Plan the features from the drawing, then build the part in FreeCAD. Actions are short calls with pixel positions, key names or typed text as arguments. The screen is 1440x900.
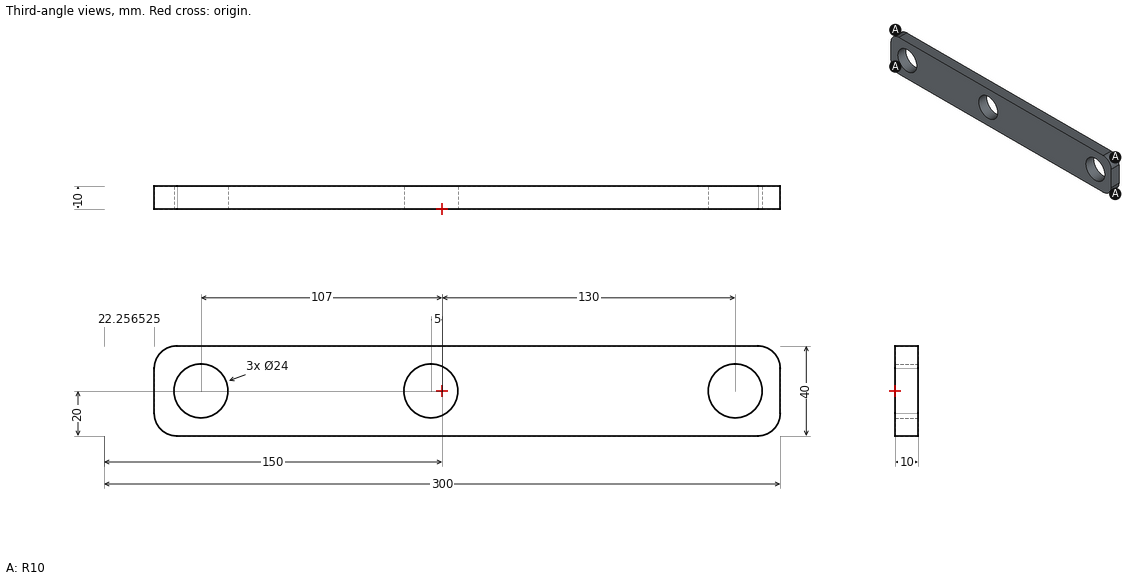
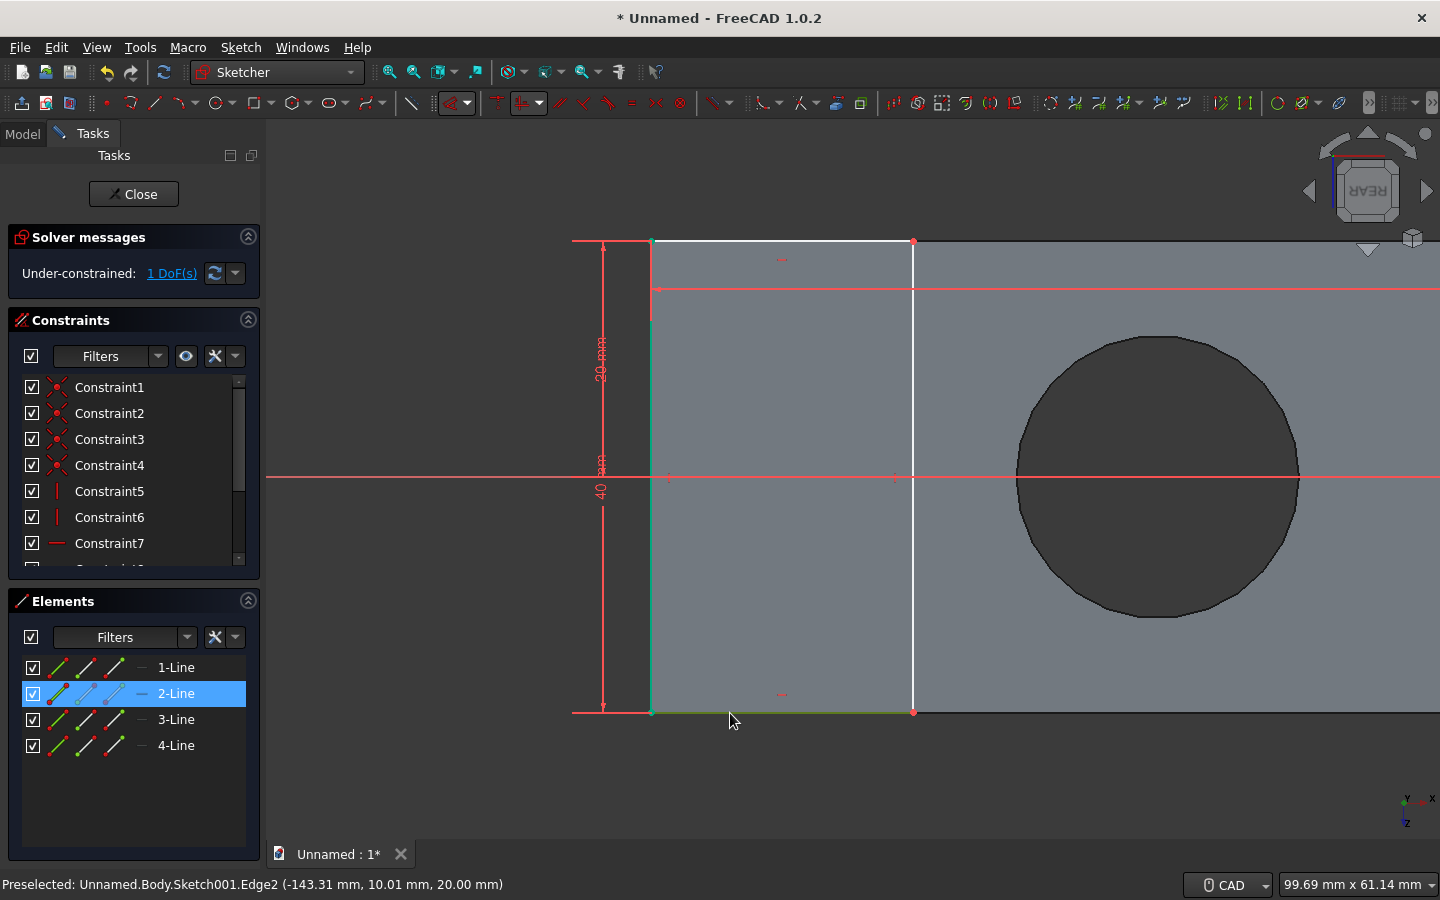
click(470, 104)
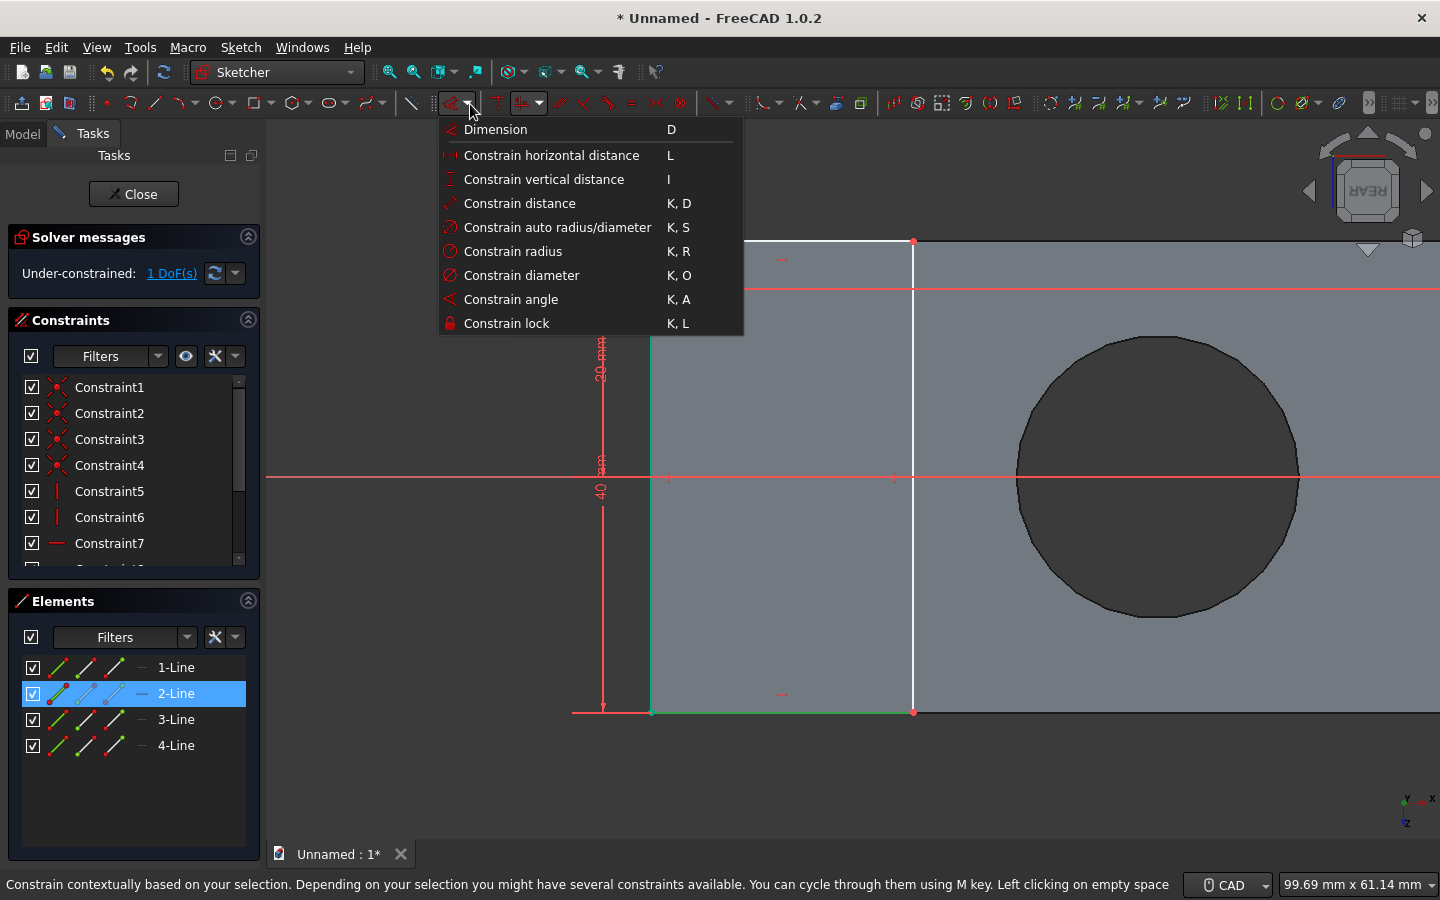
click(591, 155)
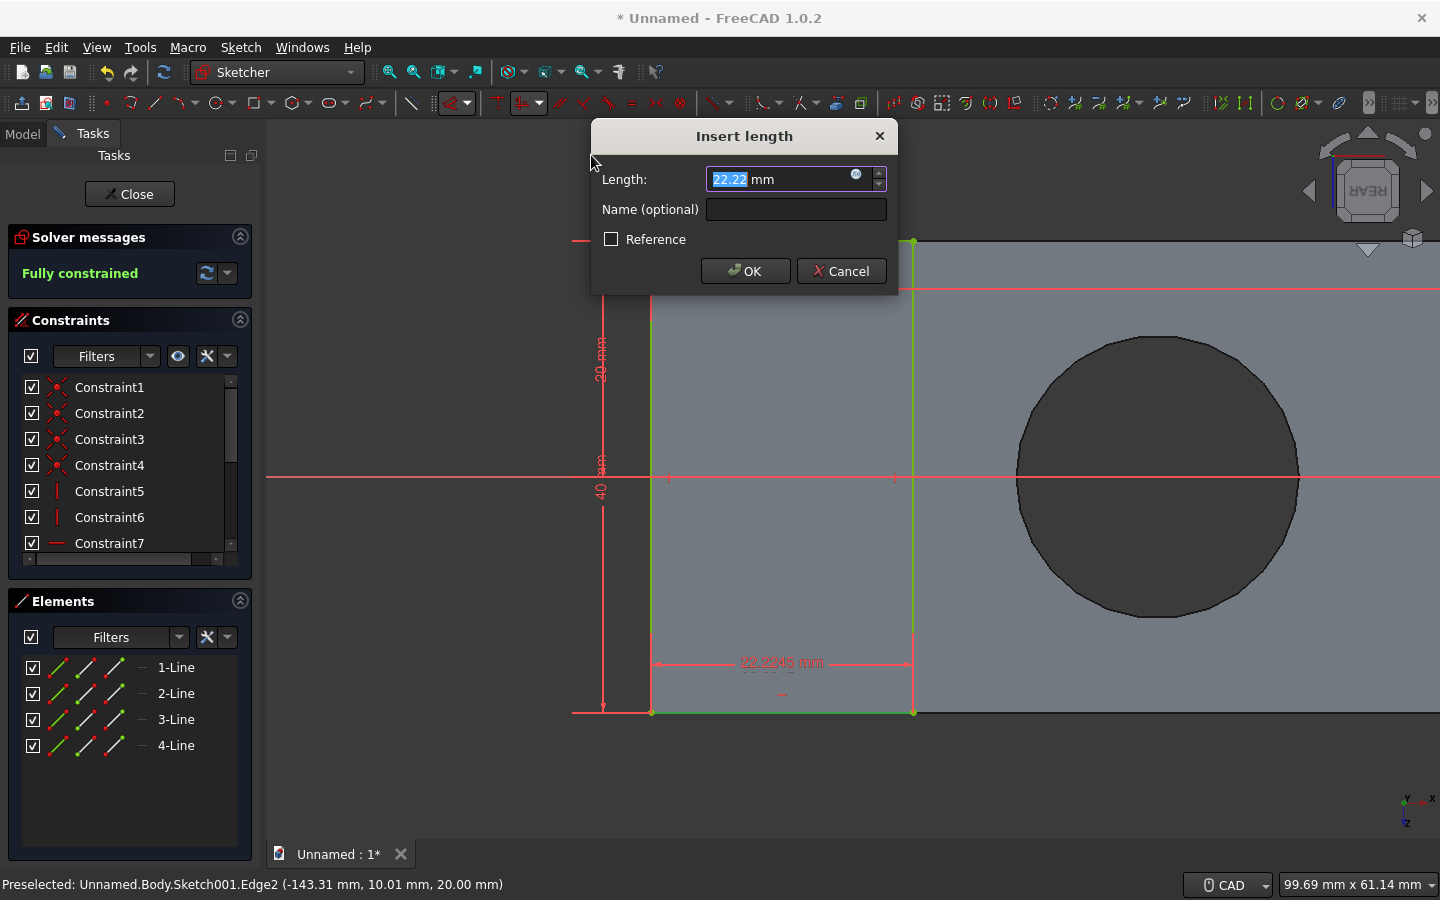
text(22.256525)
key(Return)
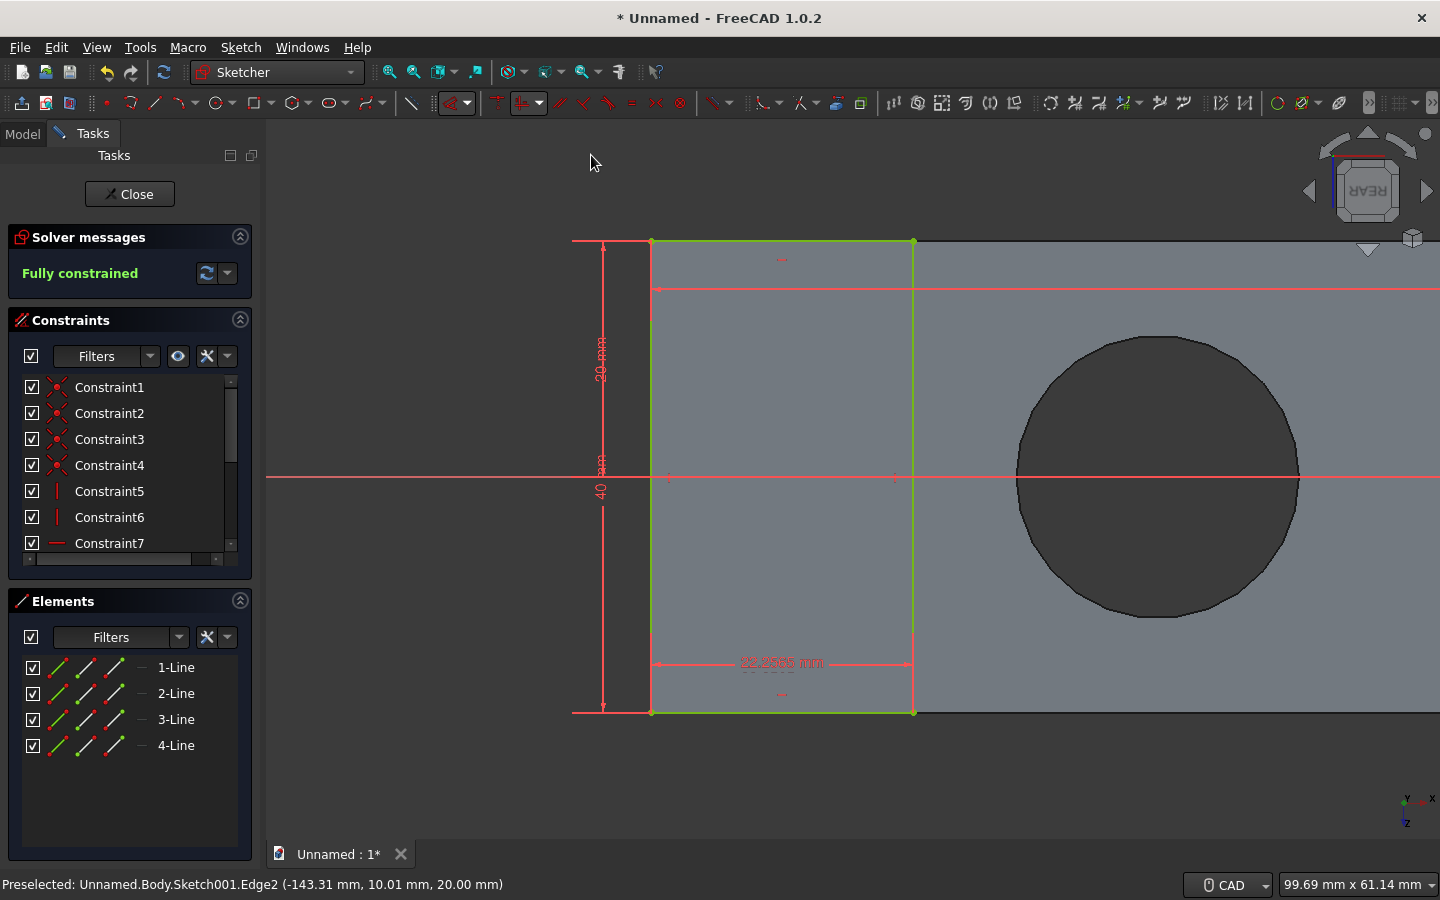
click(130, 194)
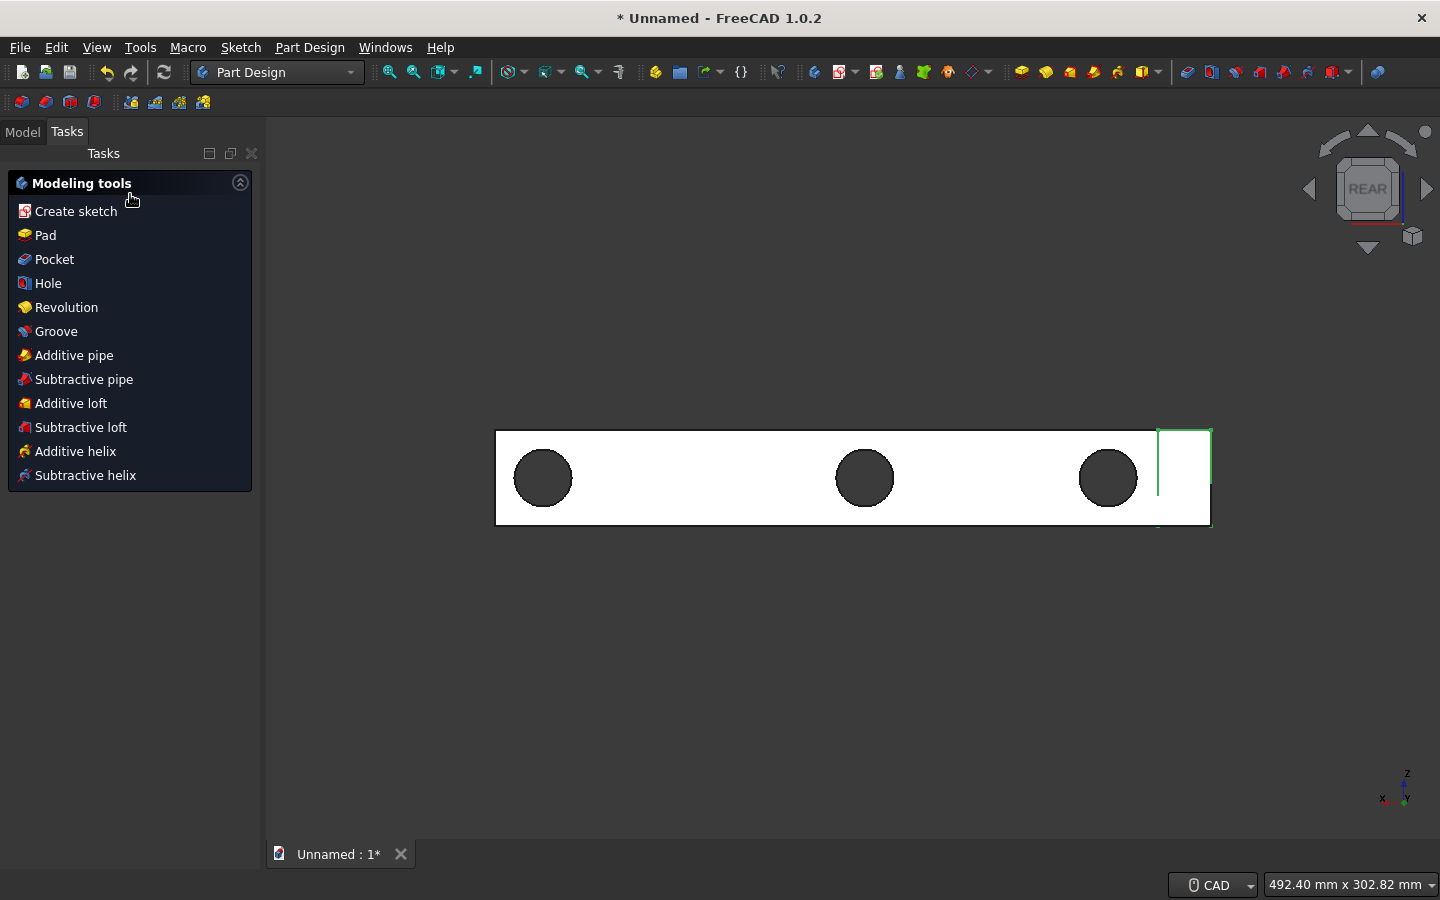
click(1188, 72)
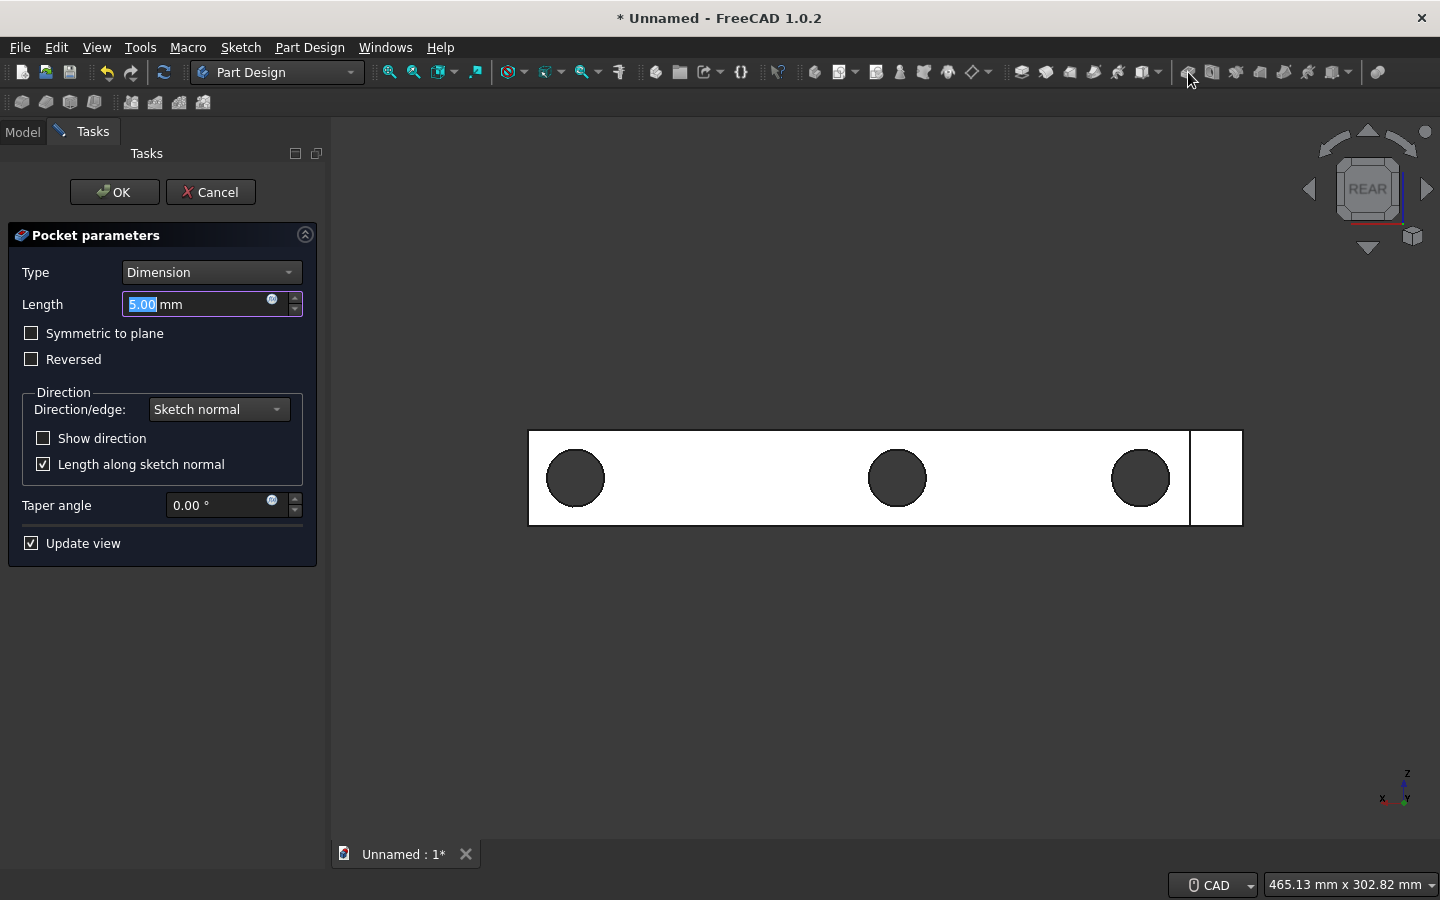
text(10)
key(Tab)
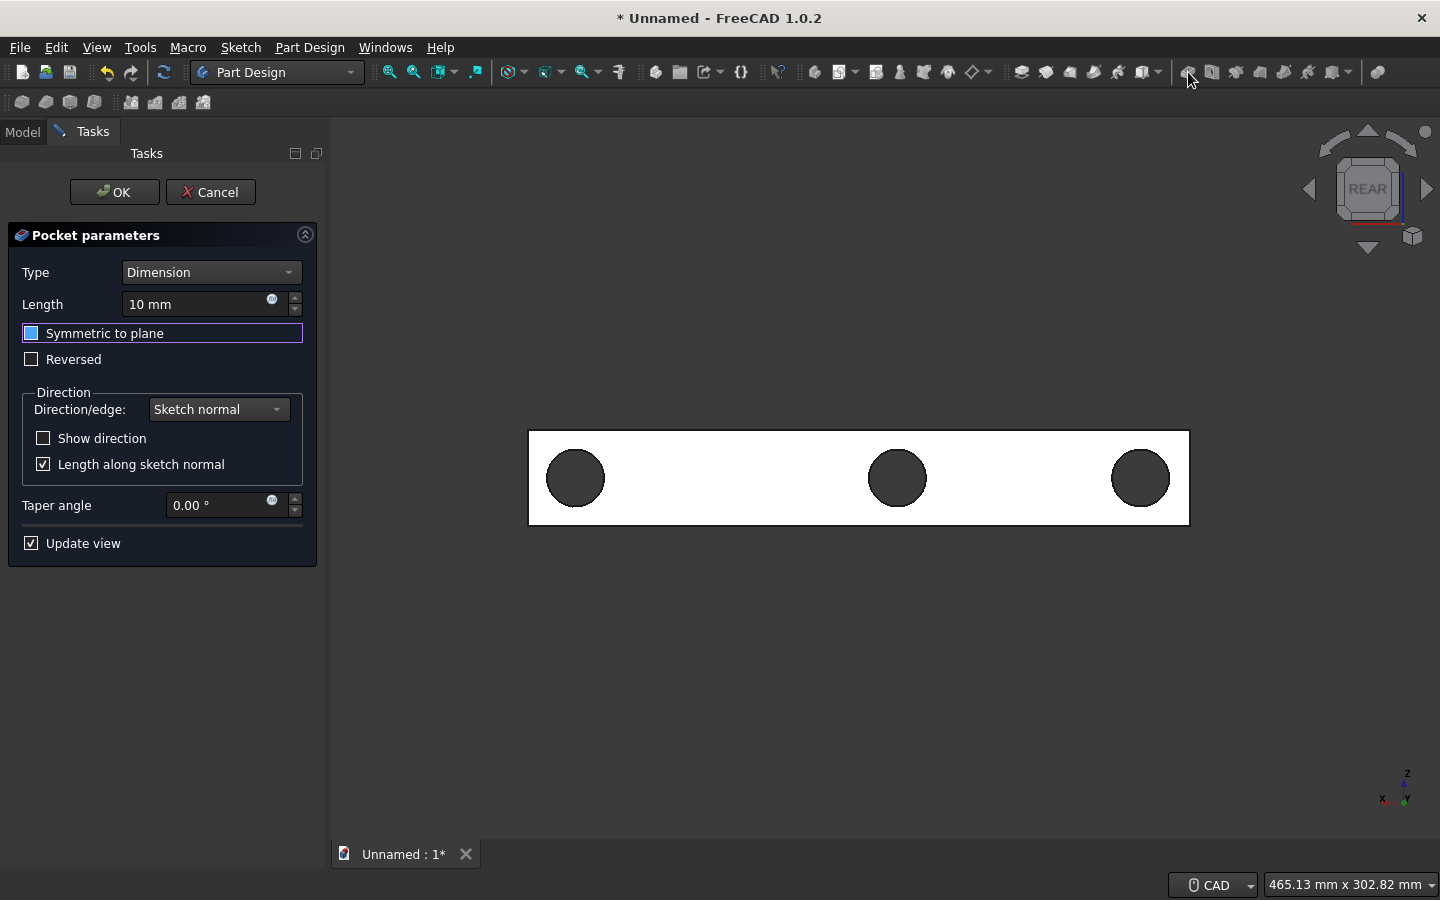
click(115, 192)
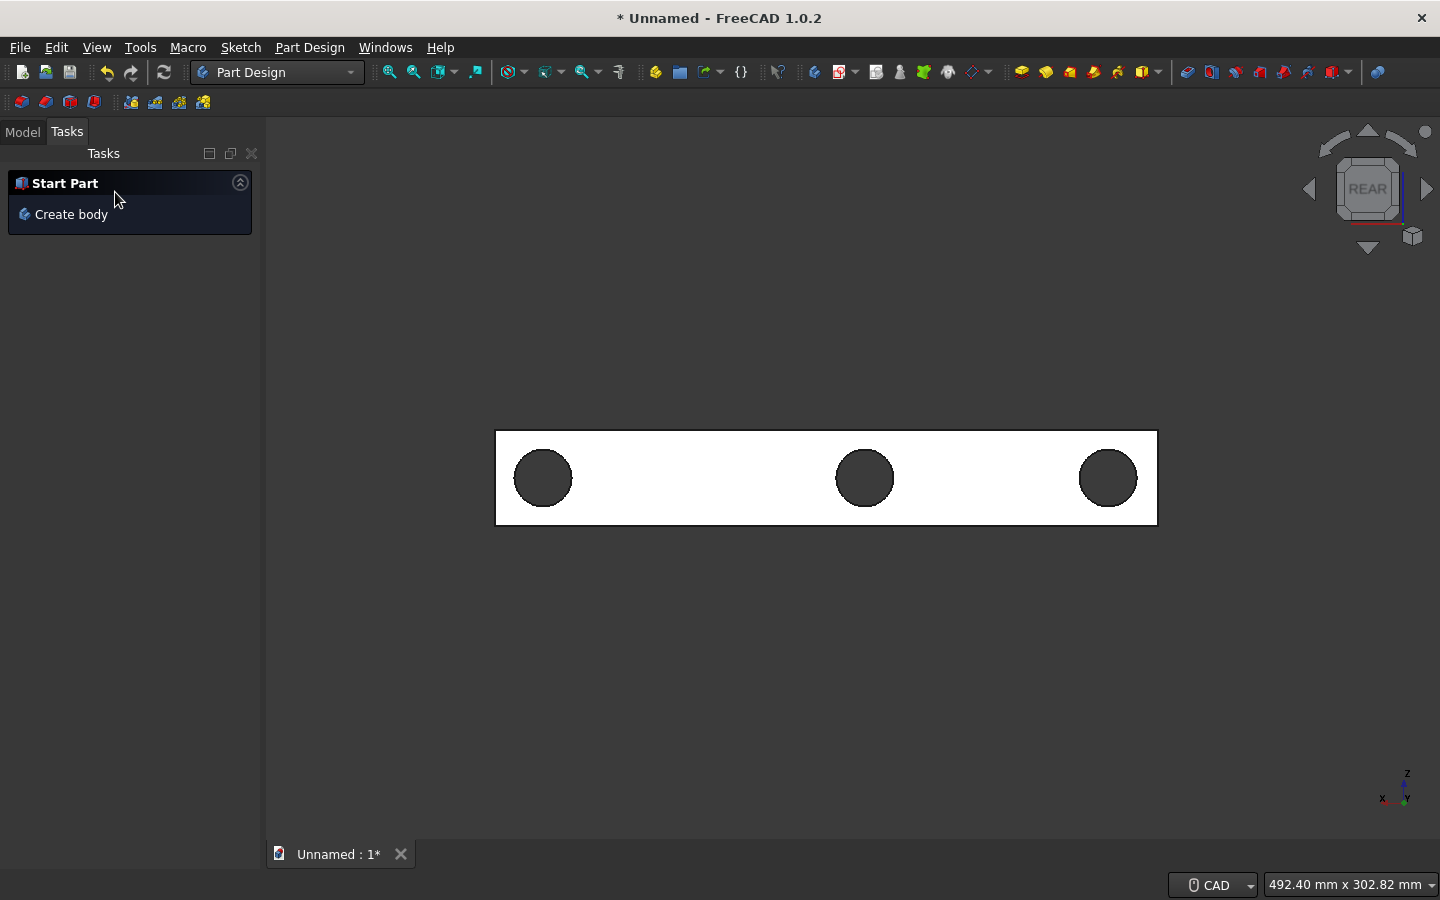
key(0)